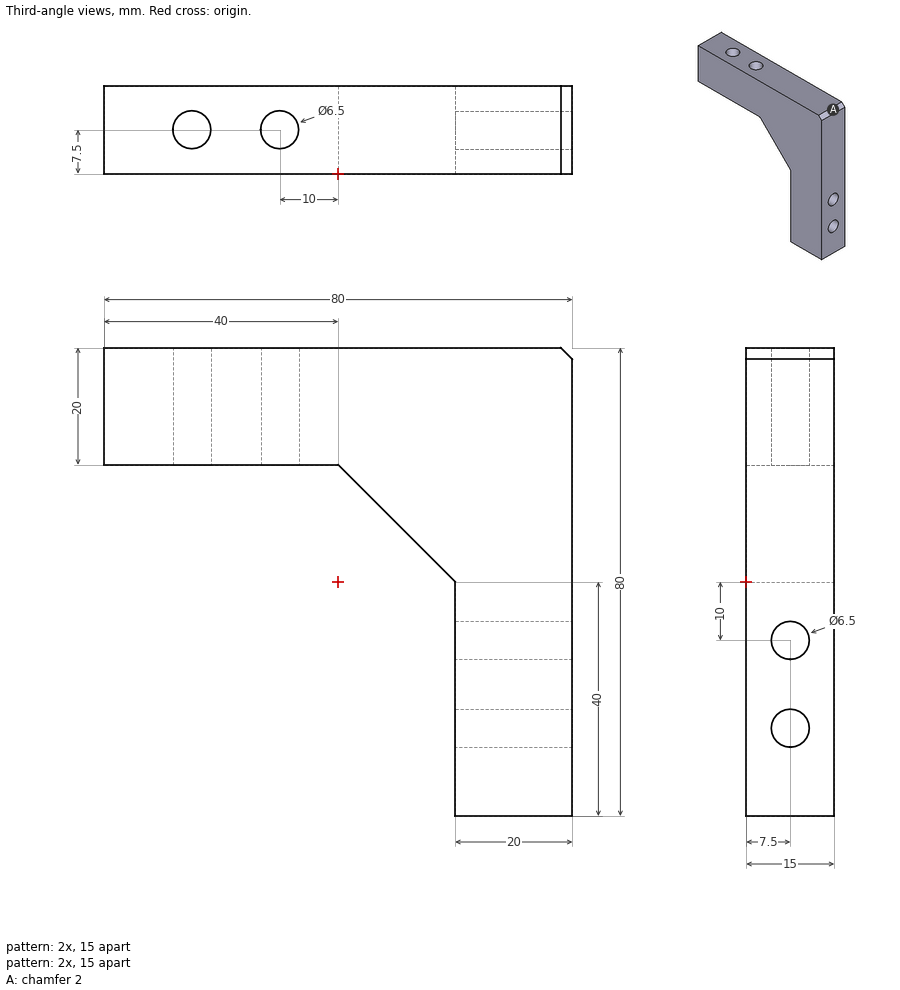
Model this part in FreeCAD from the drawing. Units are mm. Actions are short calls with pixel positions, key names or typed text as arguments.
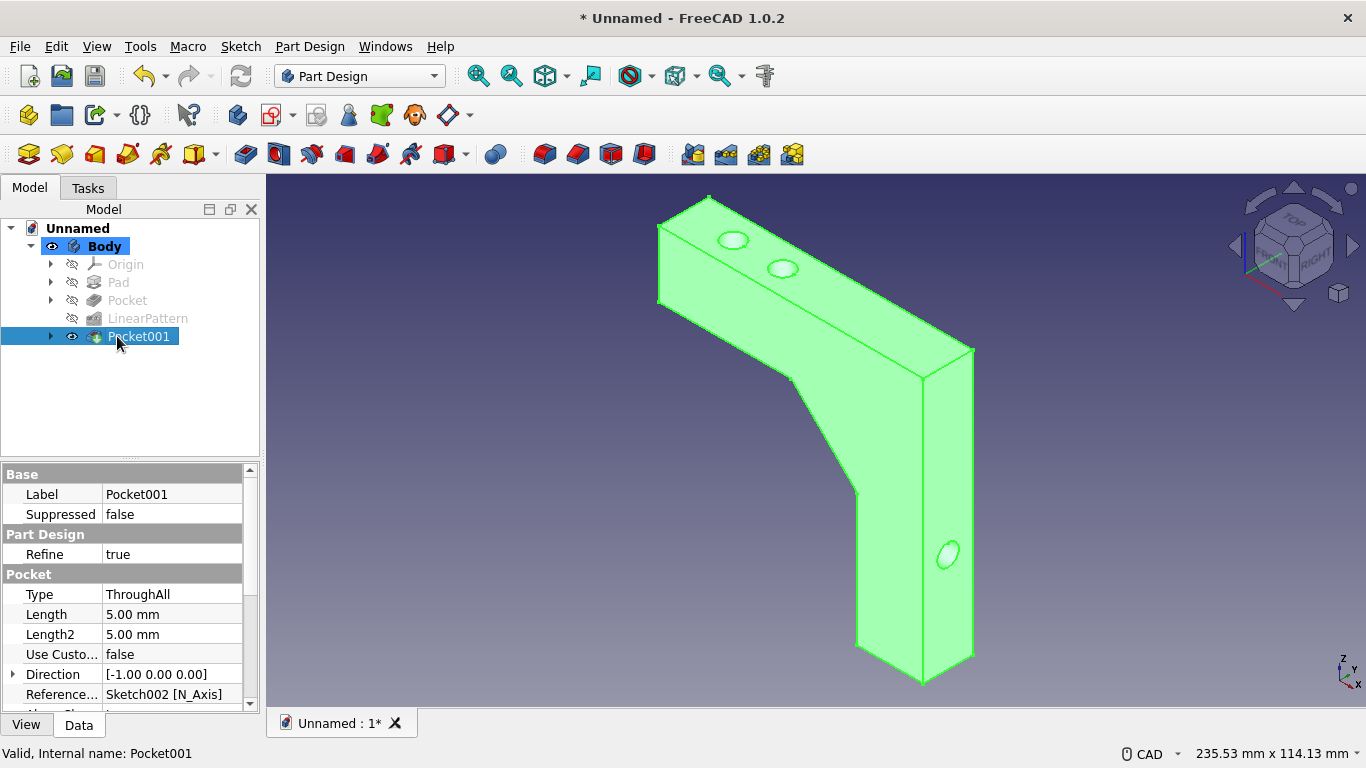
click(726, 154)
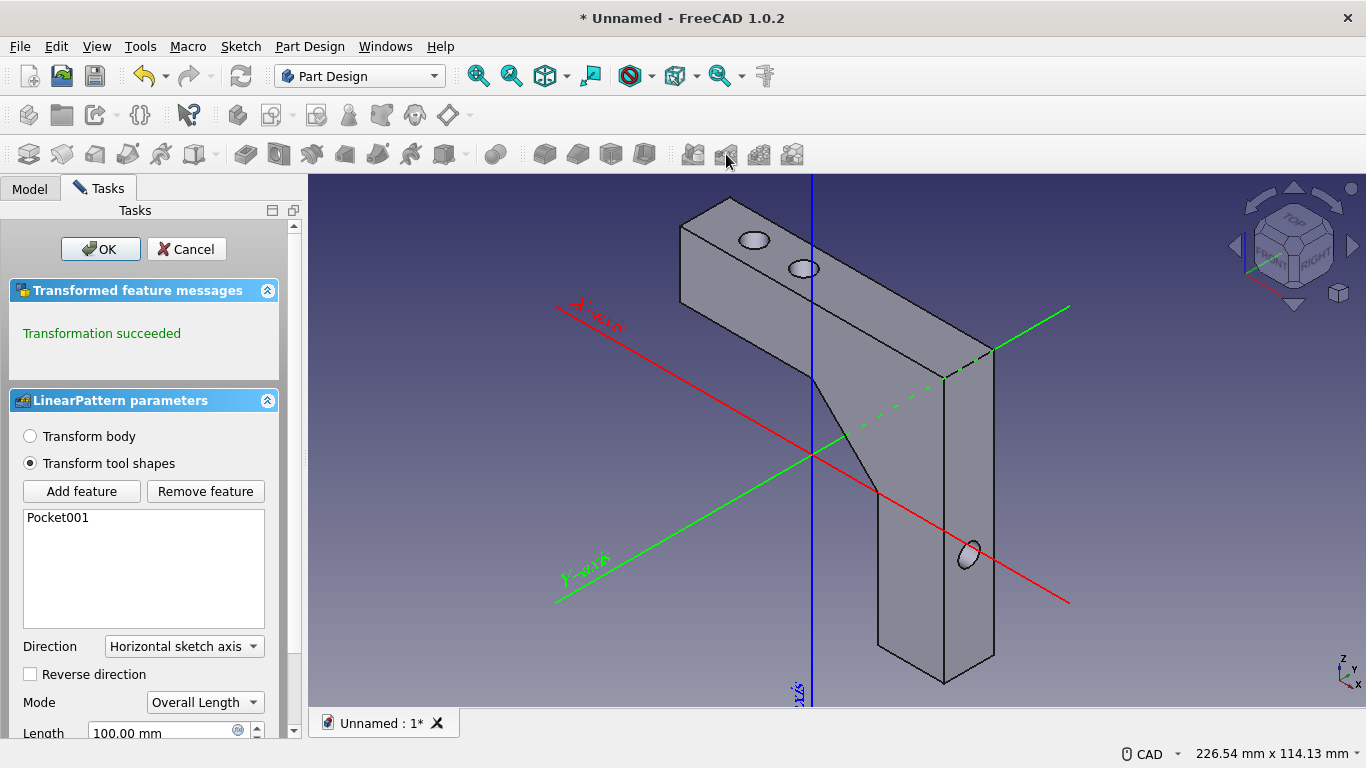
click(185, 646)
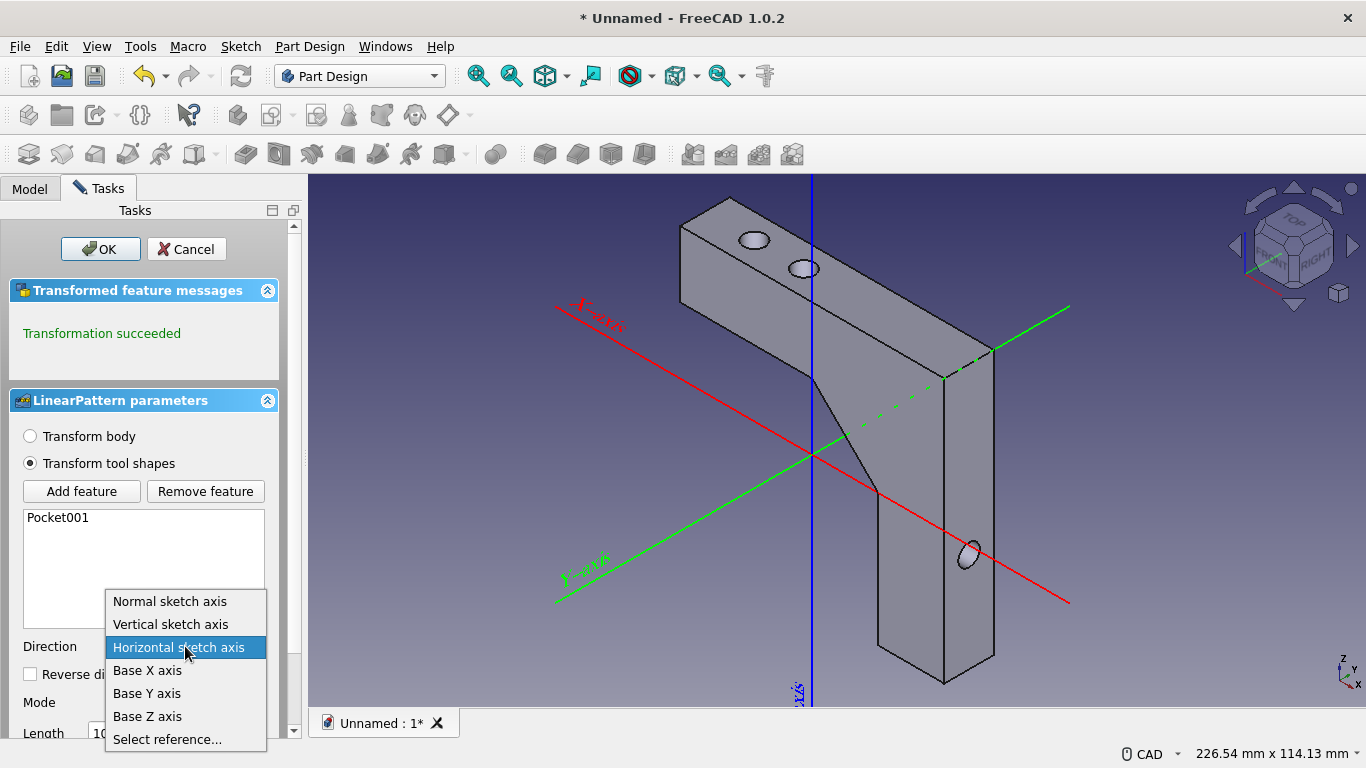
click(184, 716)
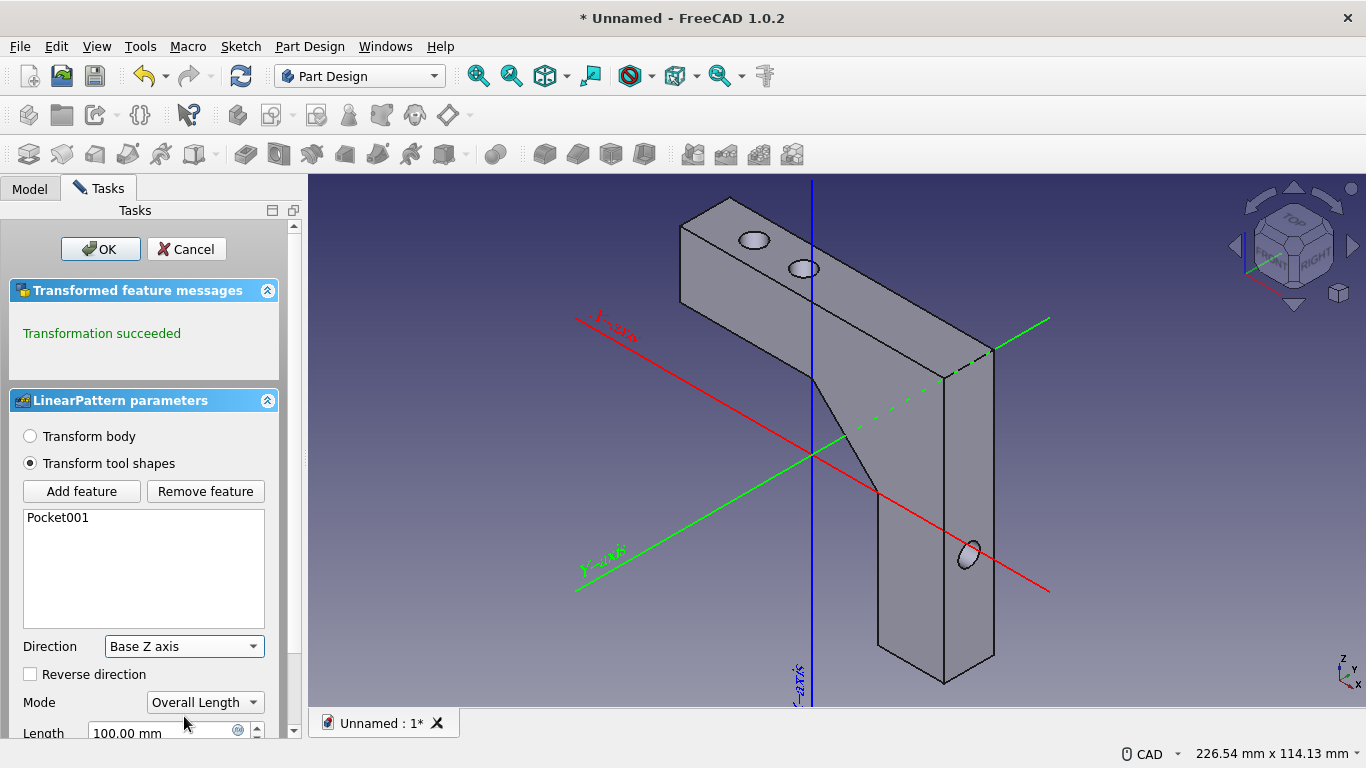
click(206, 702)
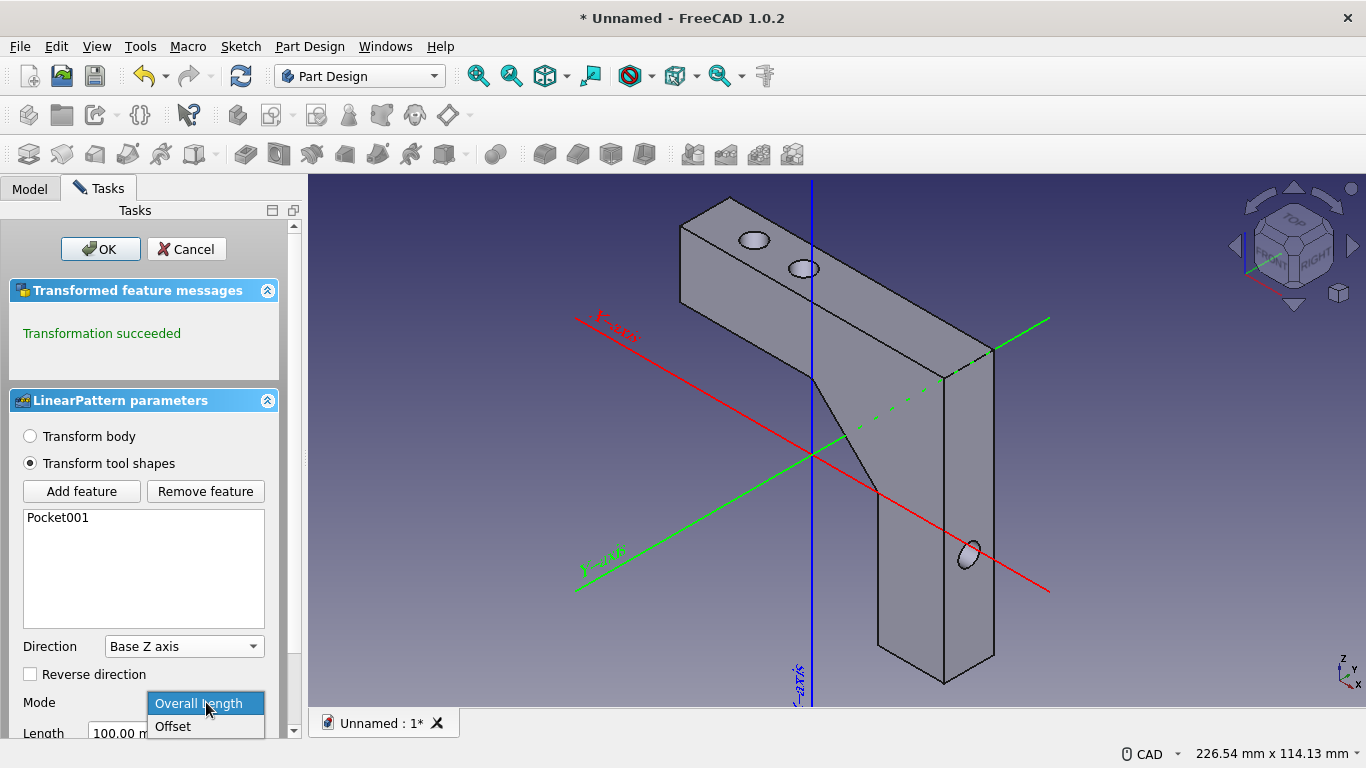
click(204, 726)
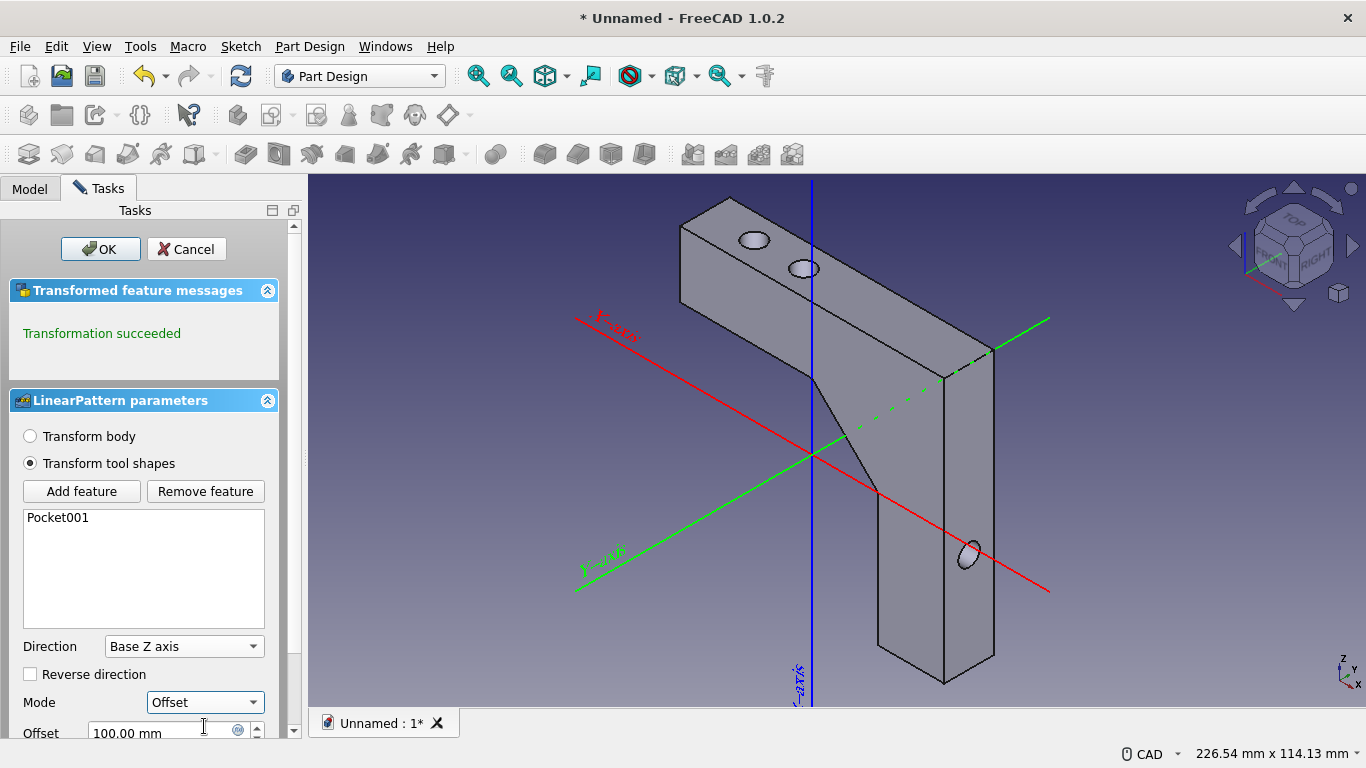
scroll(294, 479, down, 2)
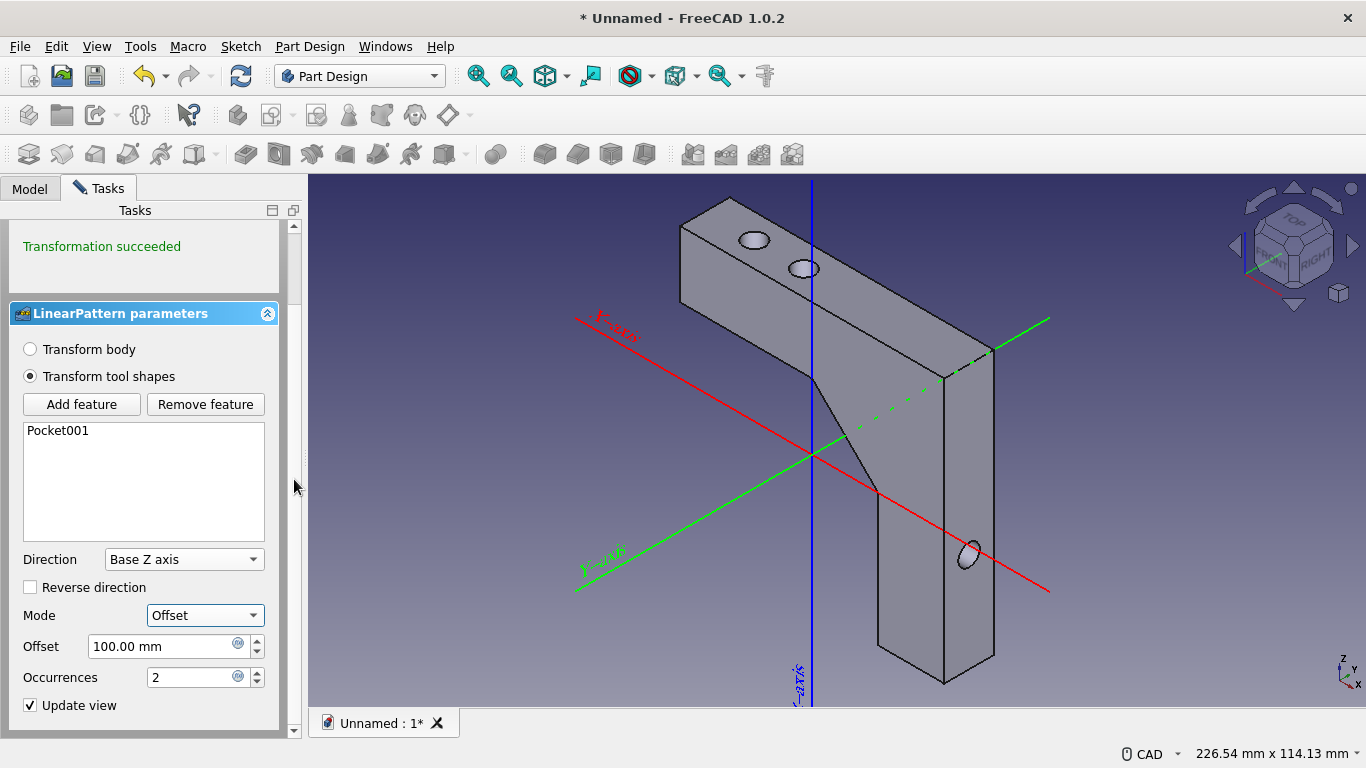
triple_click(170, 646)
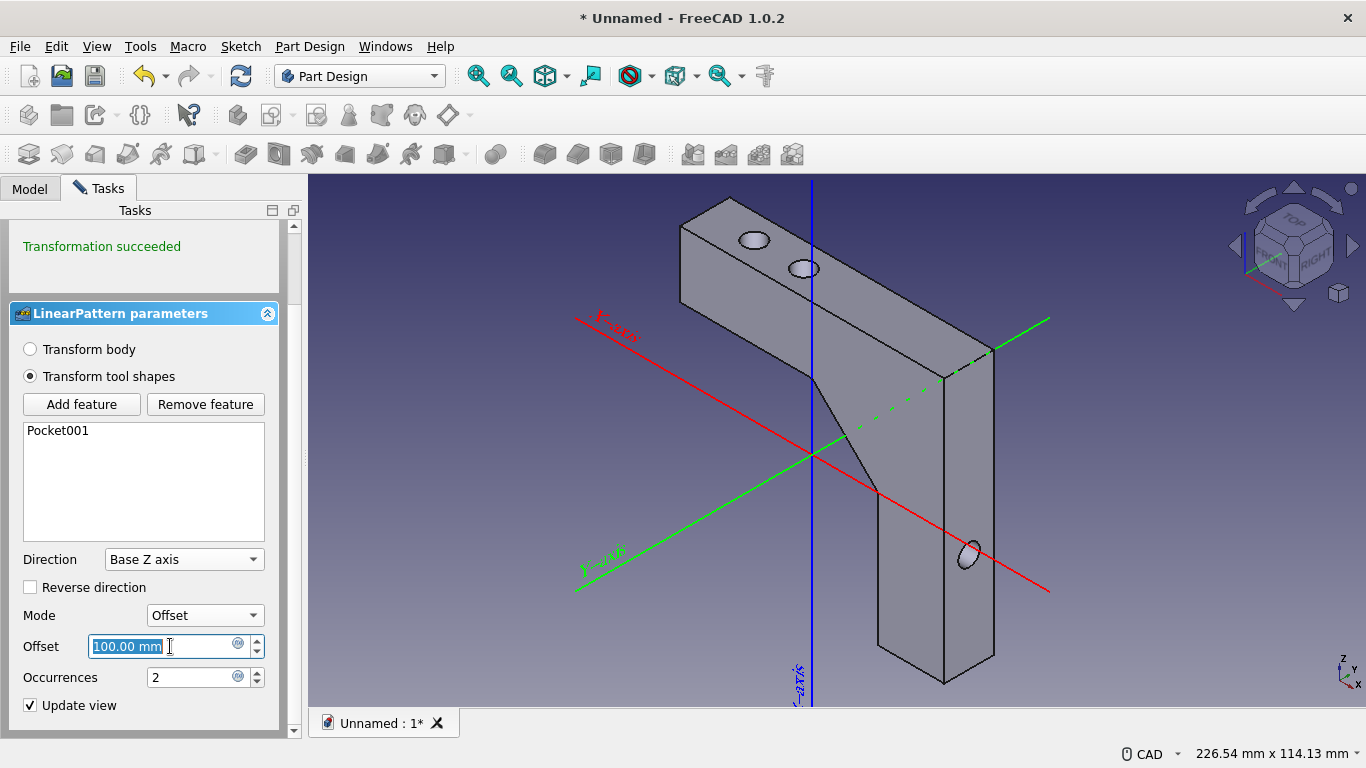
text(15)
key(Tab)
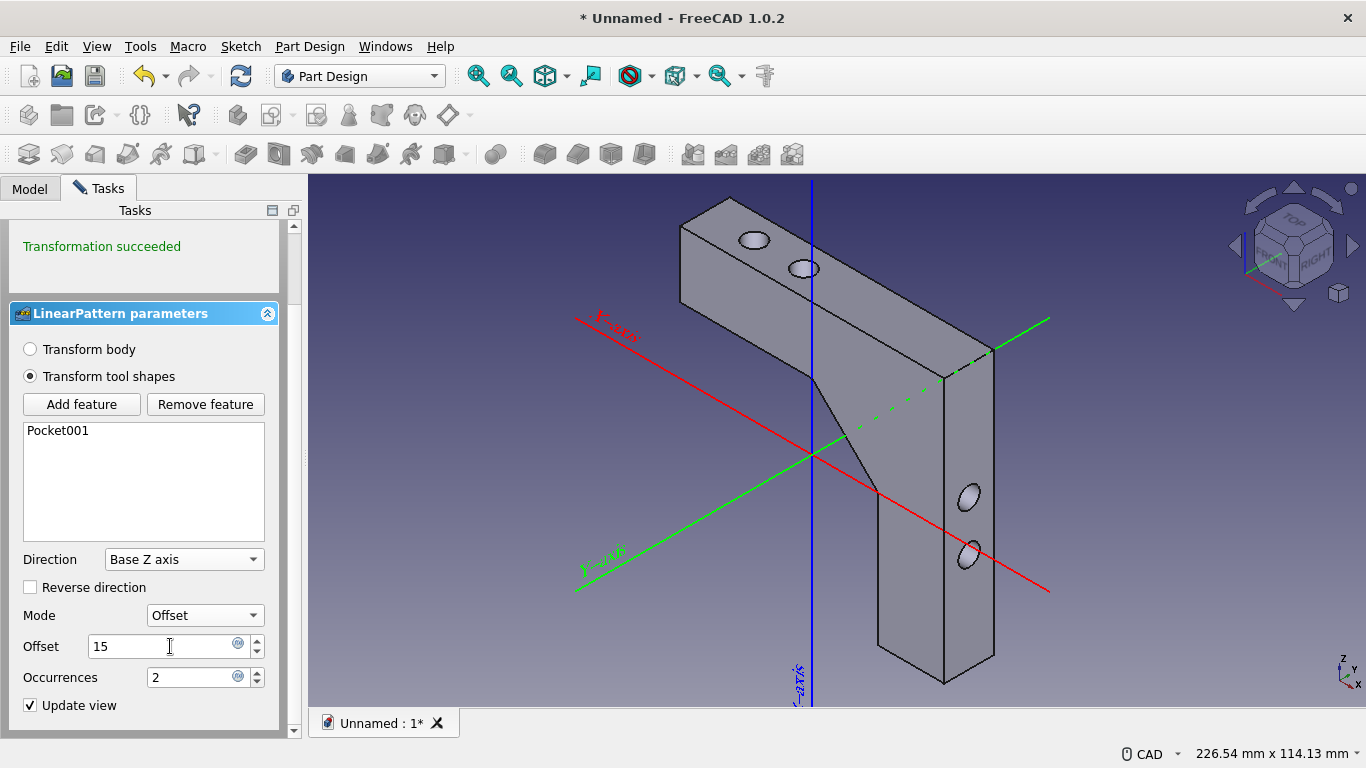
triple_click(199, 678)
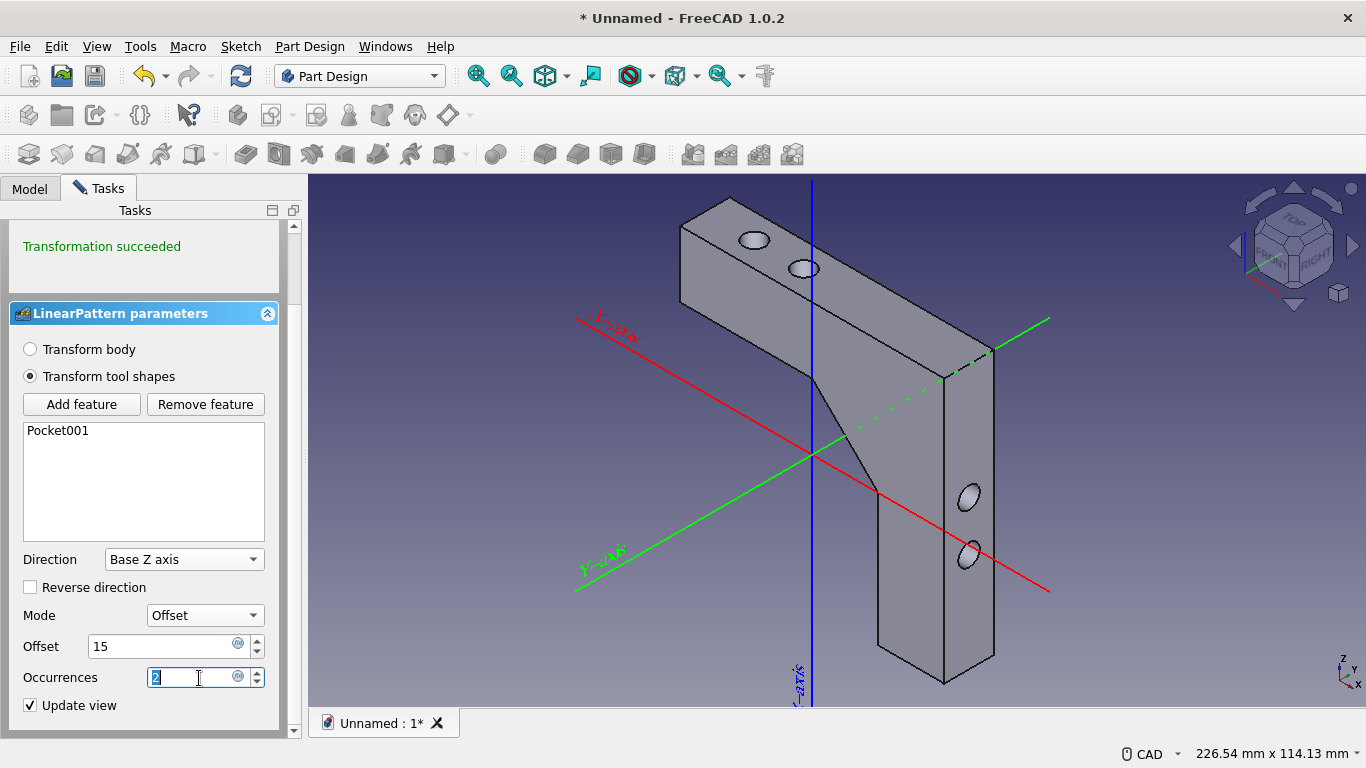
text(2)
key(Tab)